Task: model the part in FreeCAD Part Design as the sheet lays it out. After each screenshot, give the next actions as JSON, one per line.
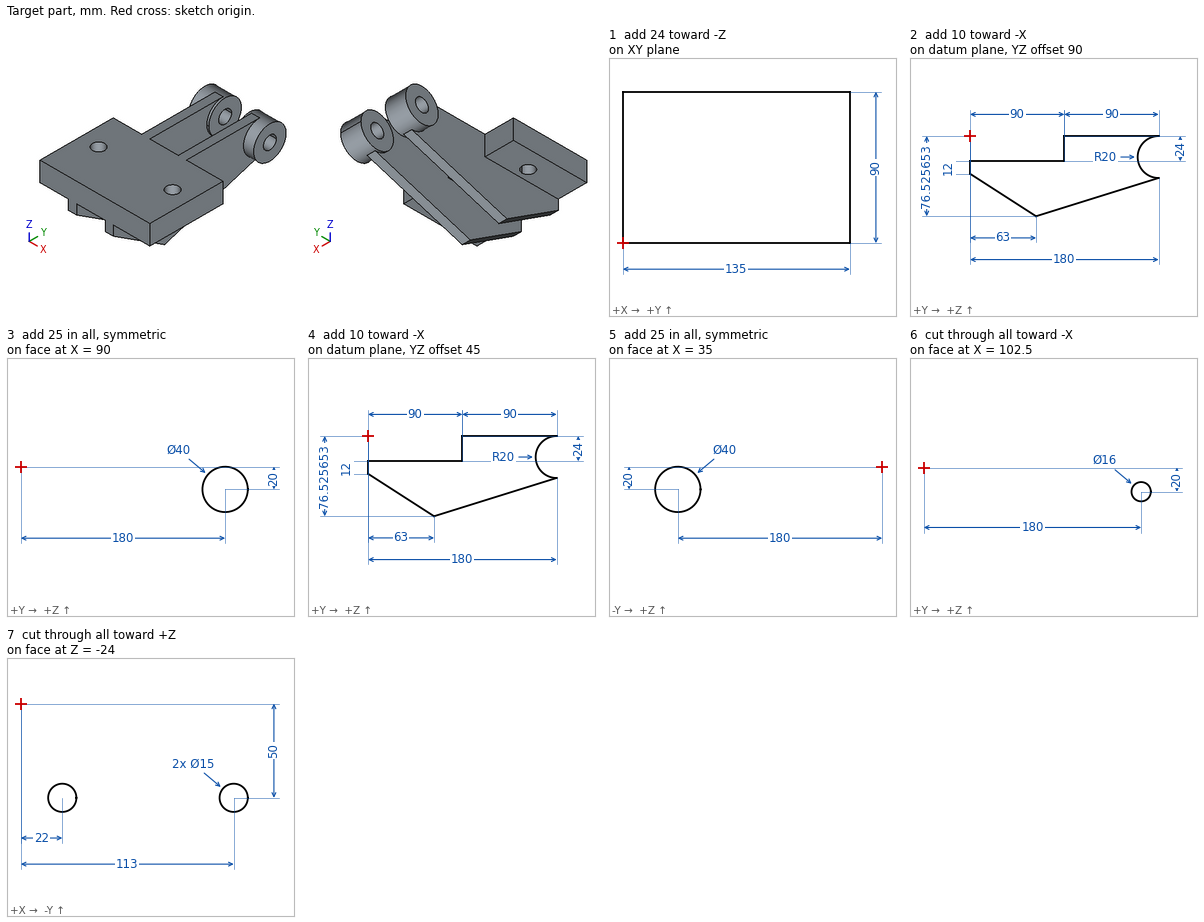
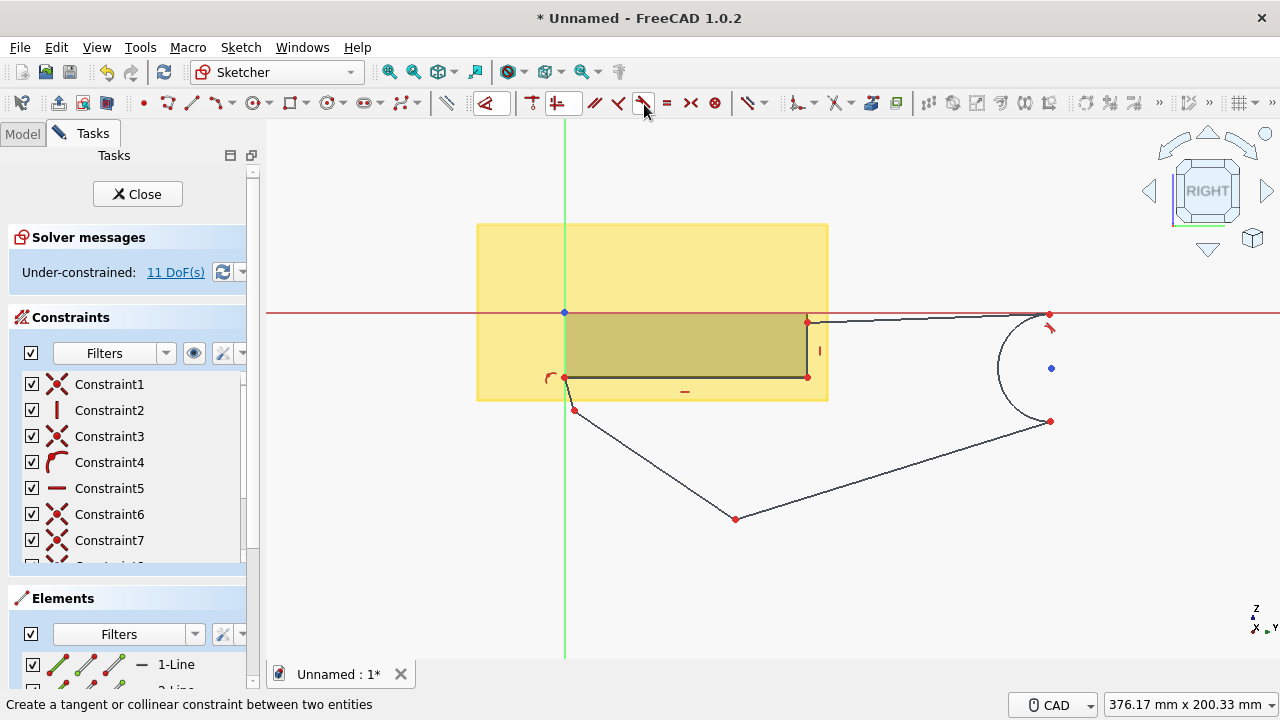
{"action": "left_click", "coordinate": [977, 317]}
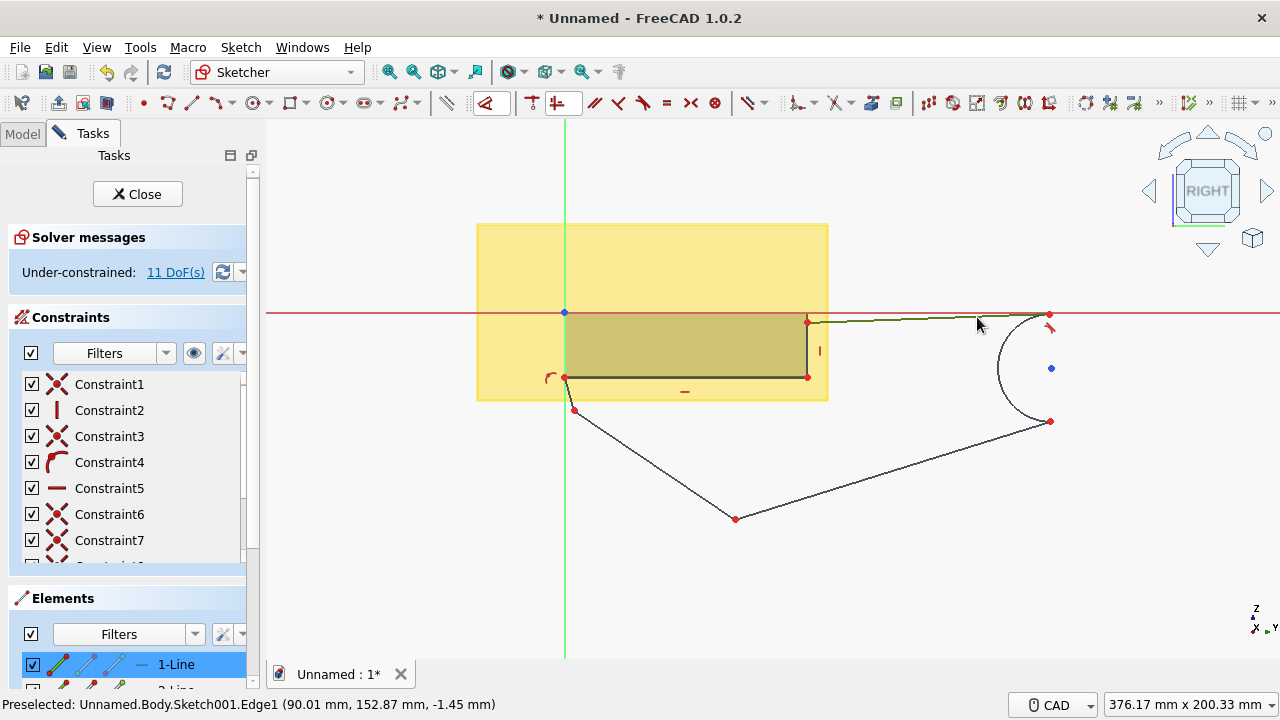
{"action": "left_click", "coordinate": [576, 104]}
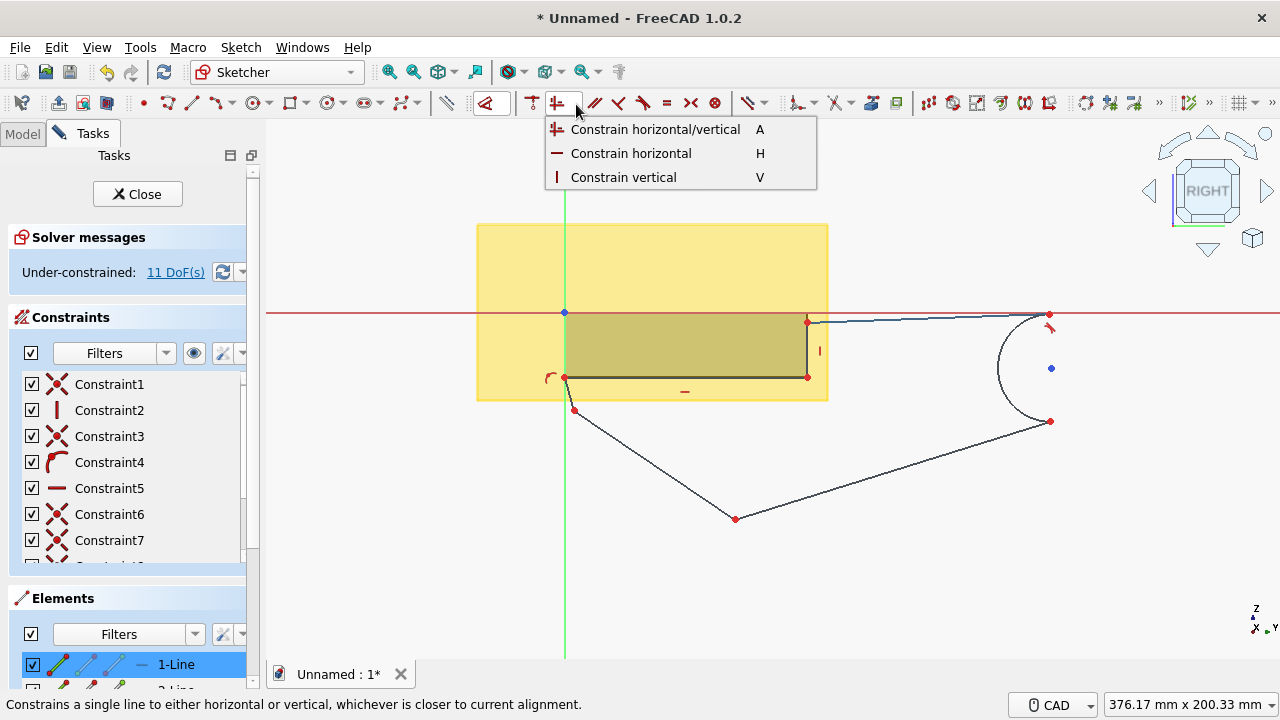
{"action": "left_click", "coordinate": [681, 153]}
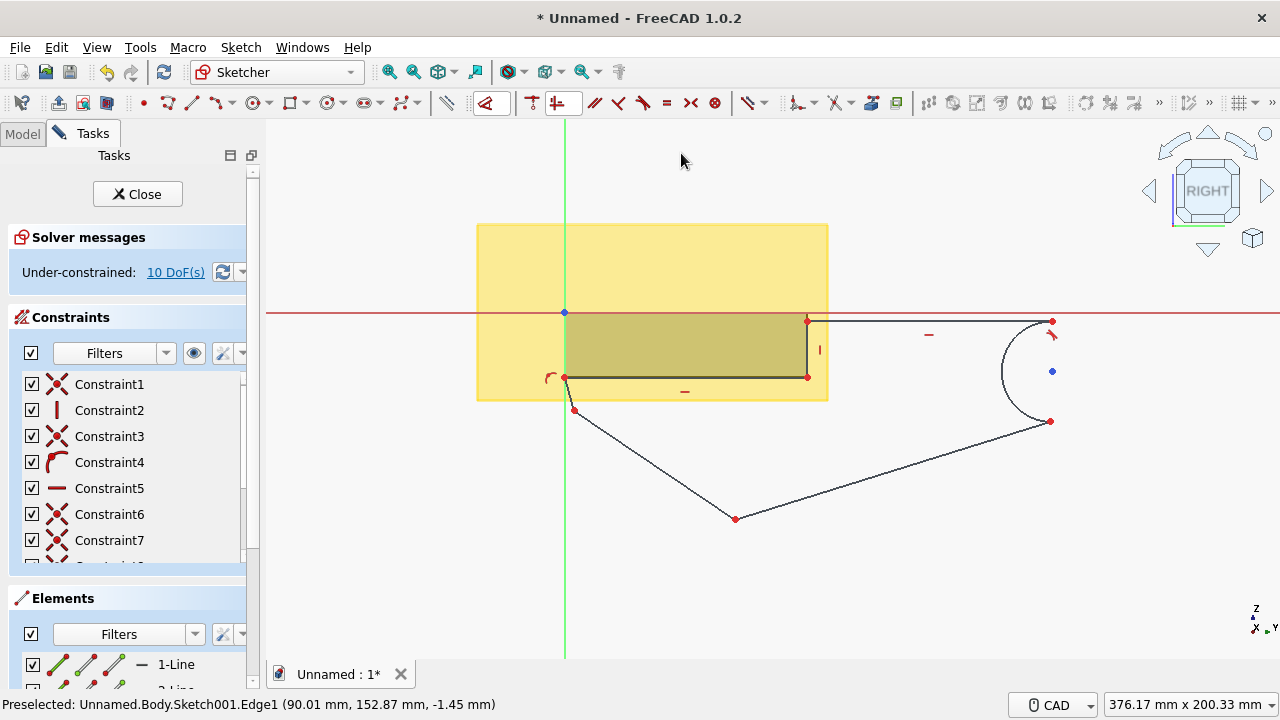
{"action": "scroll", "coordinate": [568, 388], "scroll_direction": "up", "scroll_amount": 2}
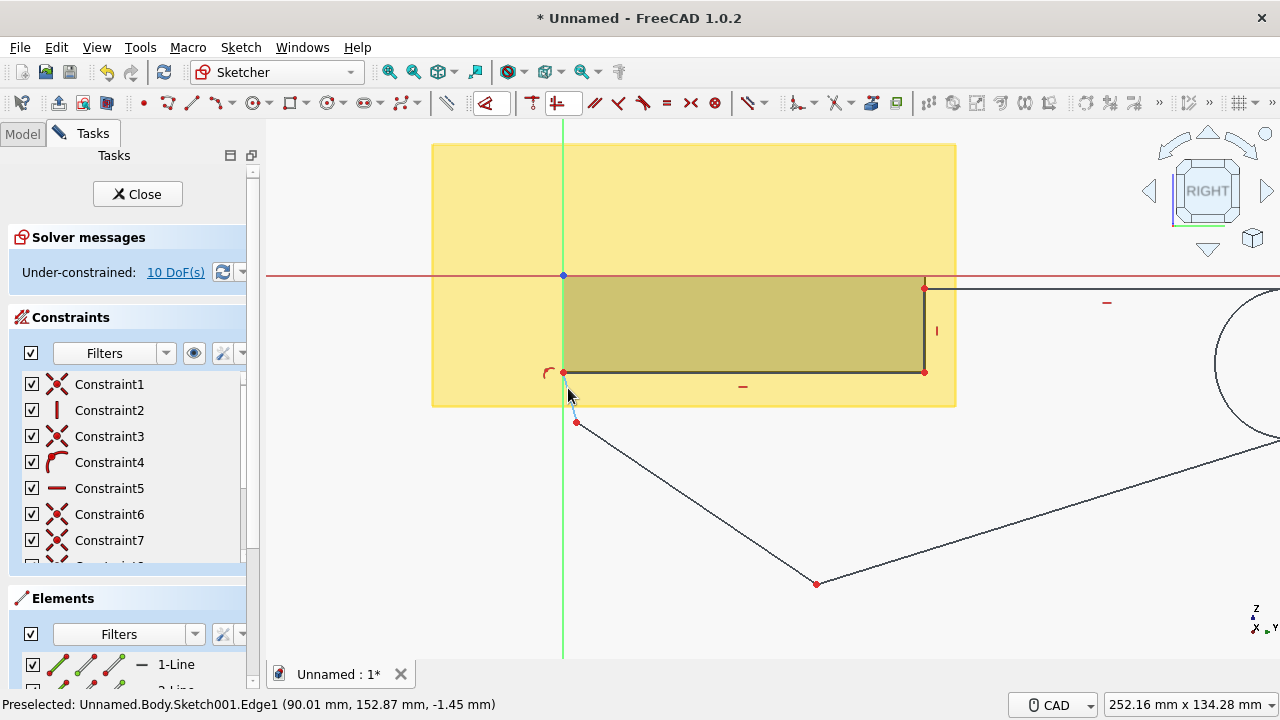
{"action": "left_click", "coordinate": [567, 388]}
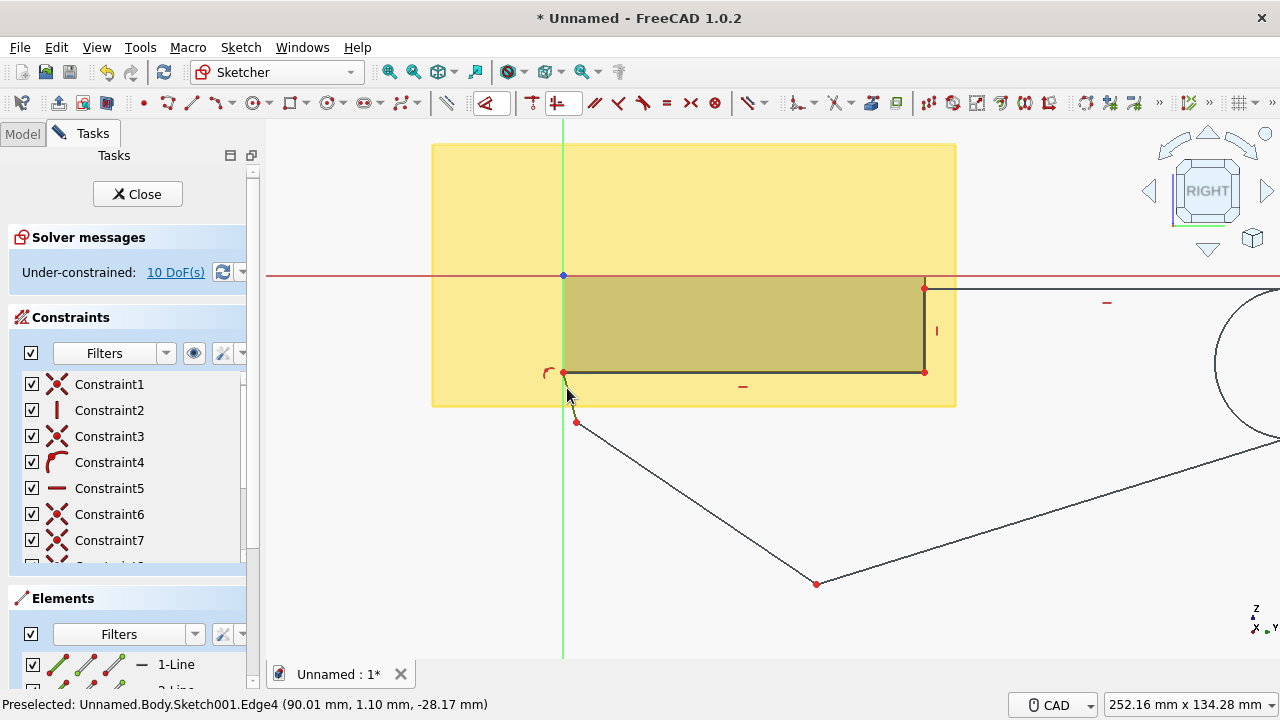
{"action": "left_click", "coordinate": [576, 104]}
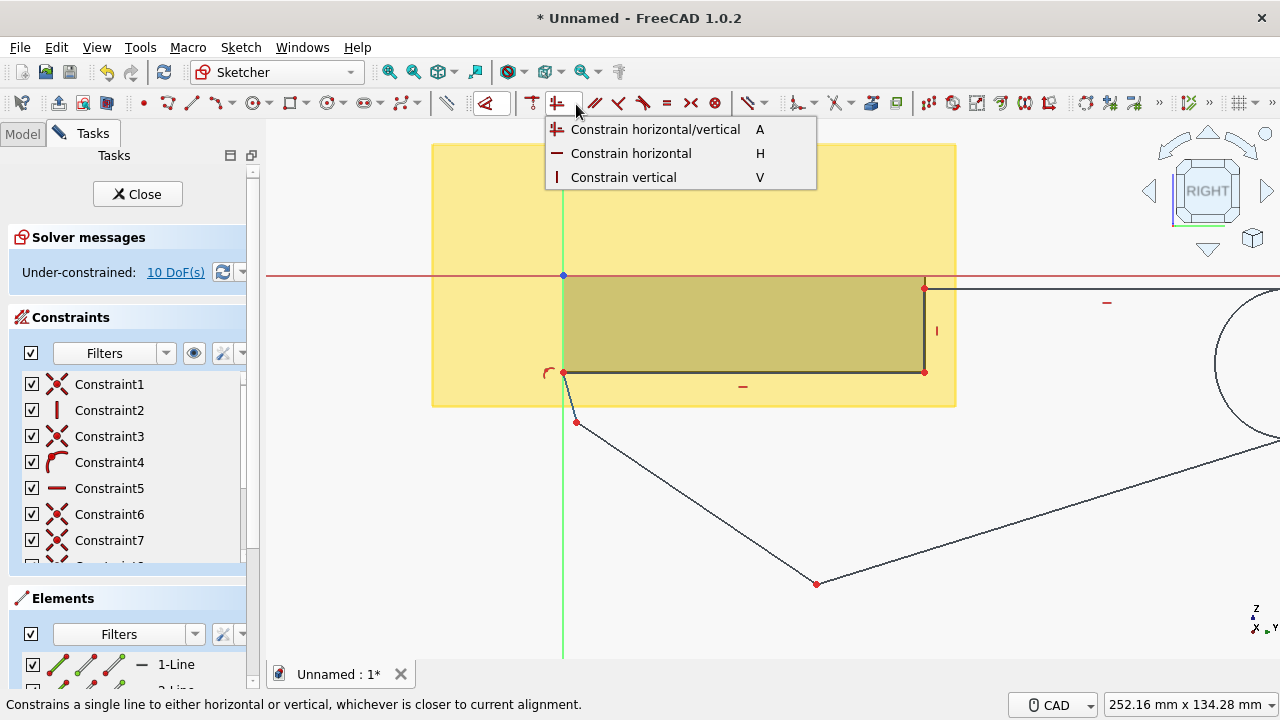
{"action": "left_click", "coordinate": [681, 177]}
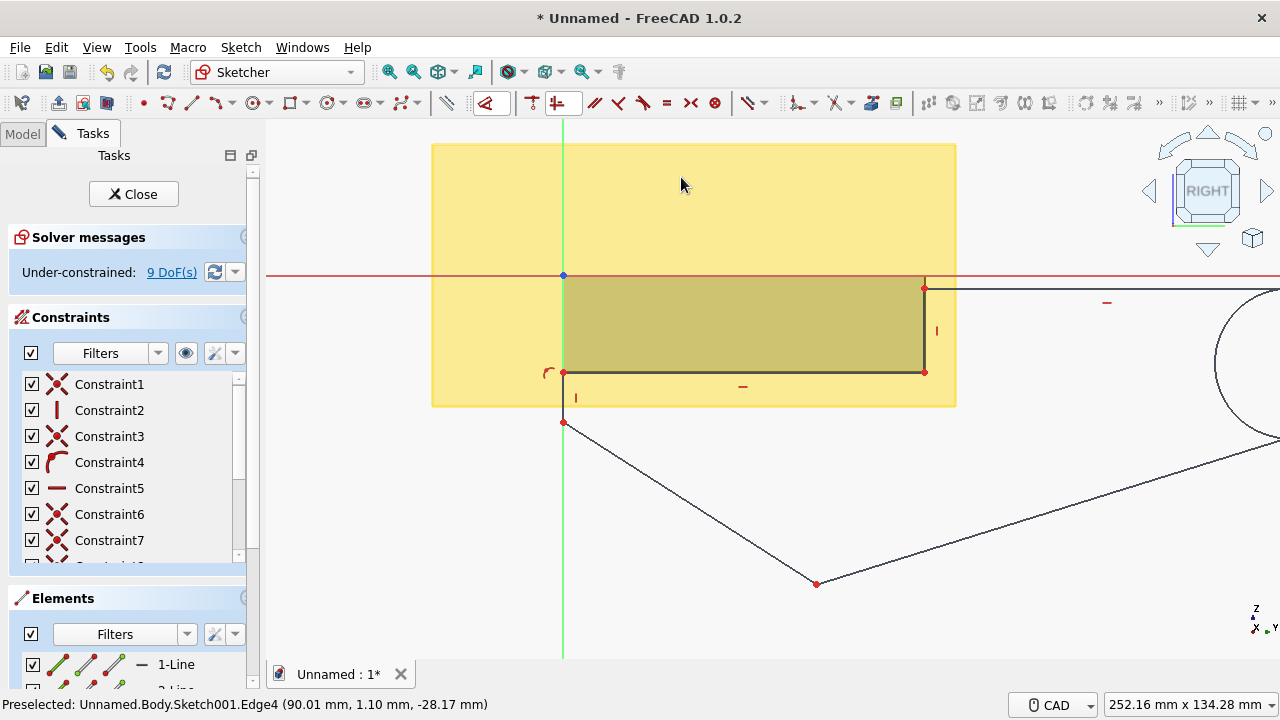
{"action": "scroll", "coordinate": [294, 307], "scroll_direction": "down", "scroll_amount": 2}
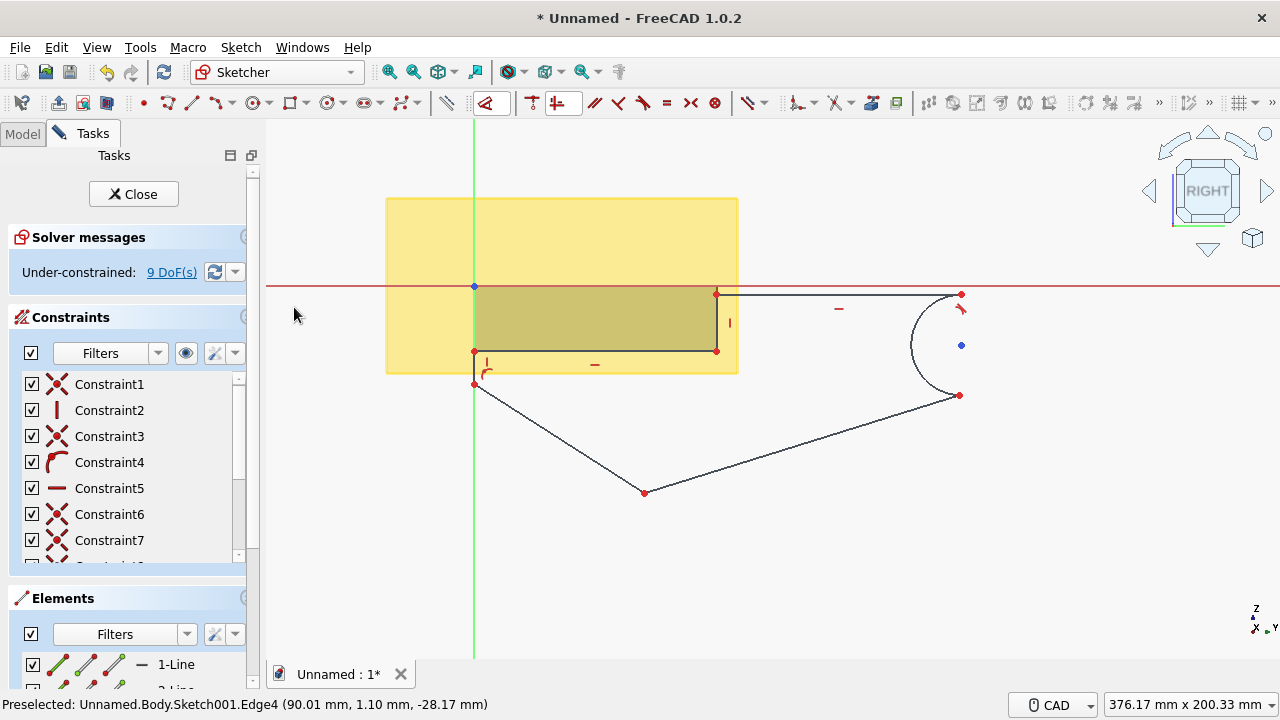
{"action": "left_click", "coordinate": [921, 315]}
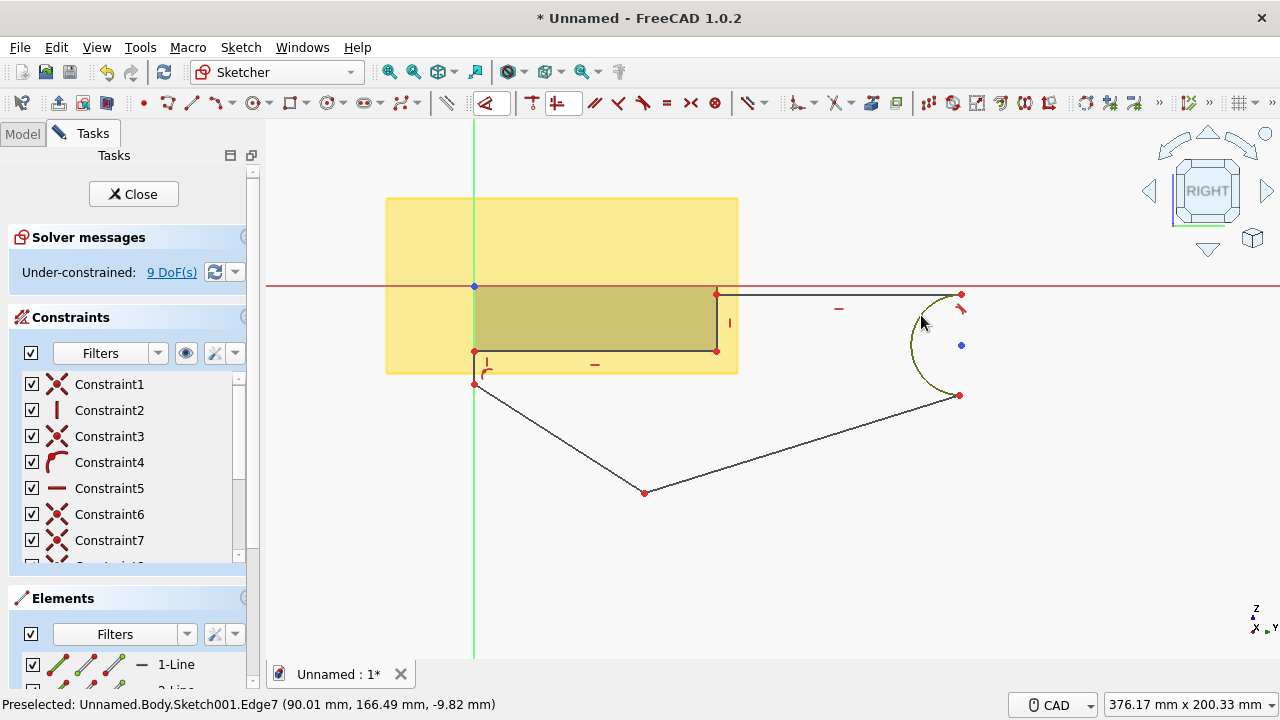
{"action": "key", "text": "k r"}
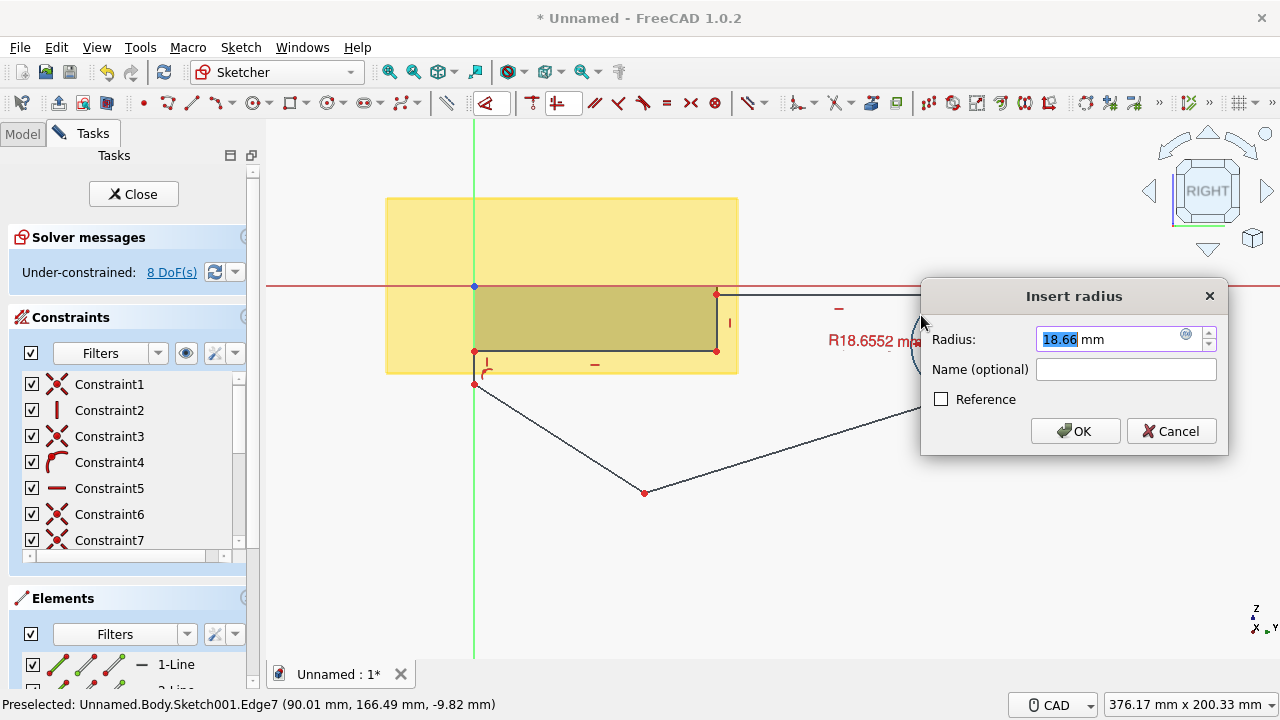
{"action": "type", "text": "20"}
{"action": "key", "text": "Return"}